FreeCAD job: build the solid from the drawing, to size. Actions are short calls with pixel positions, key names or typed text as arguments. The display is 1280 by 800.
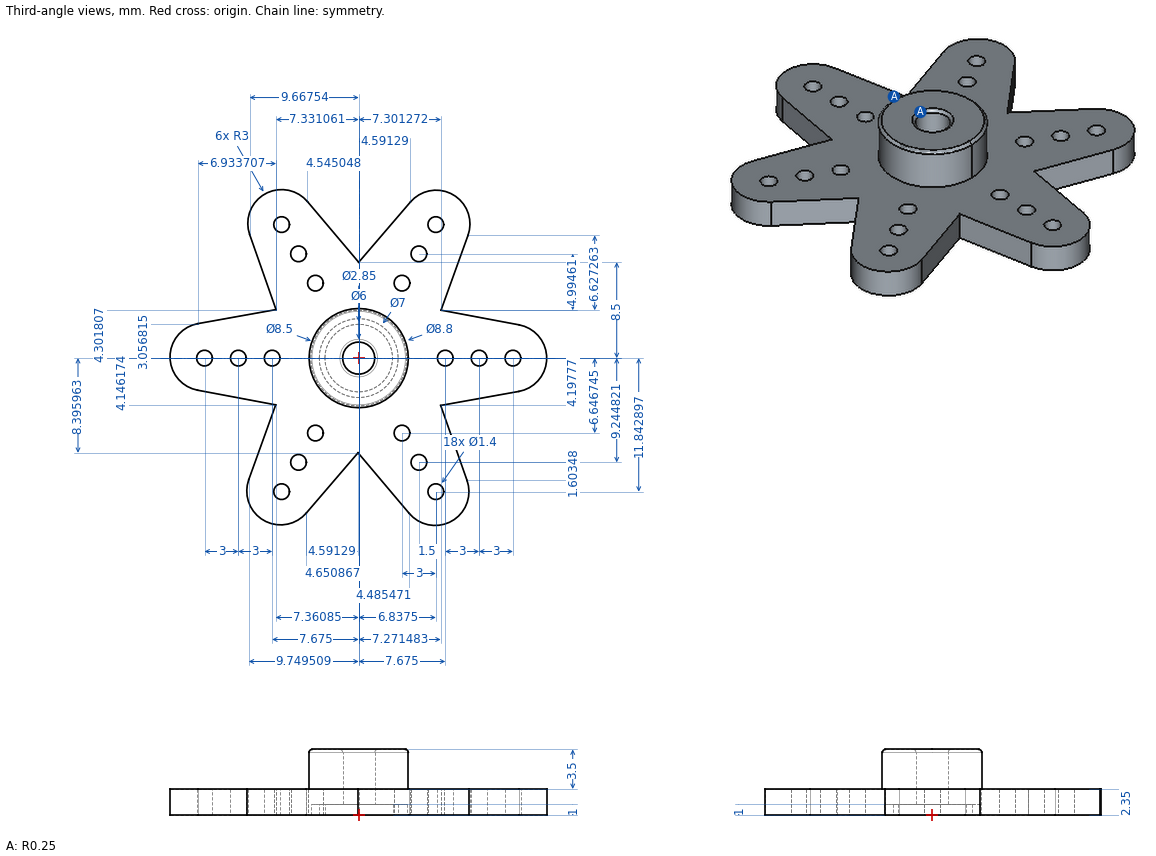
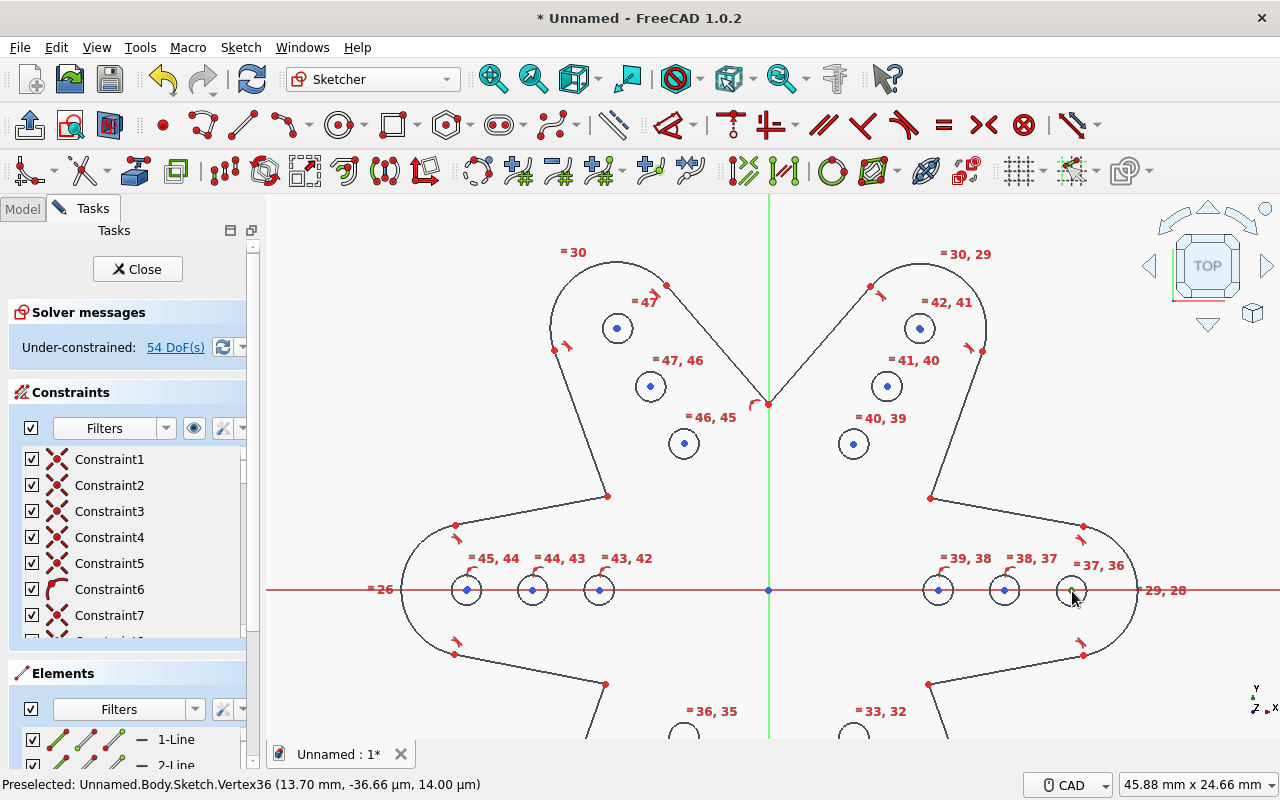
click(353, 590)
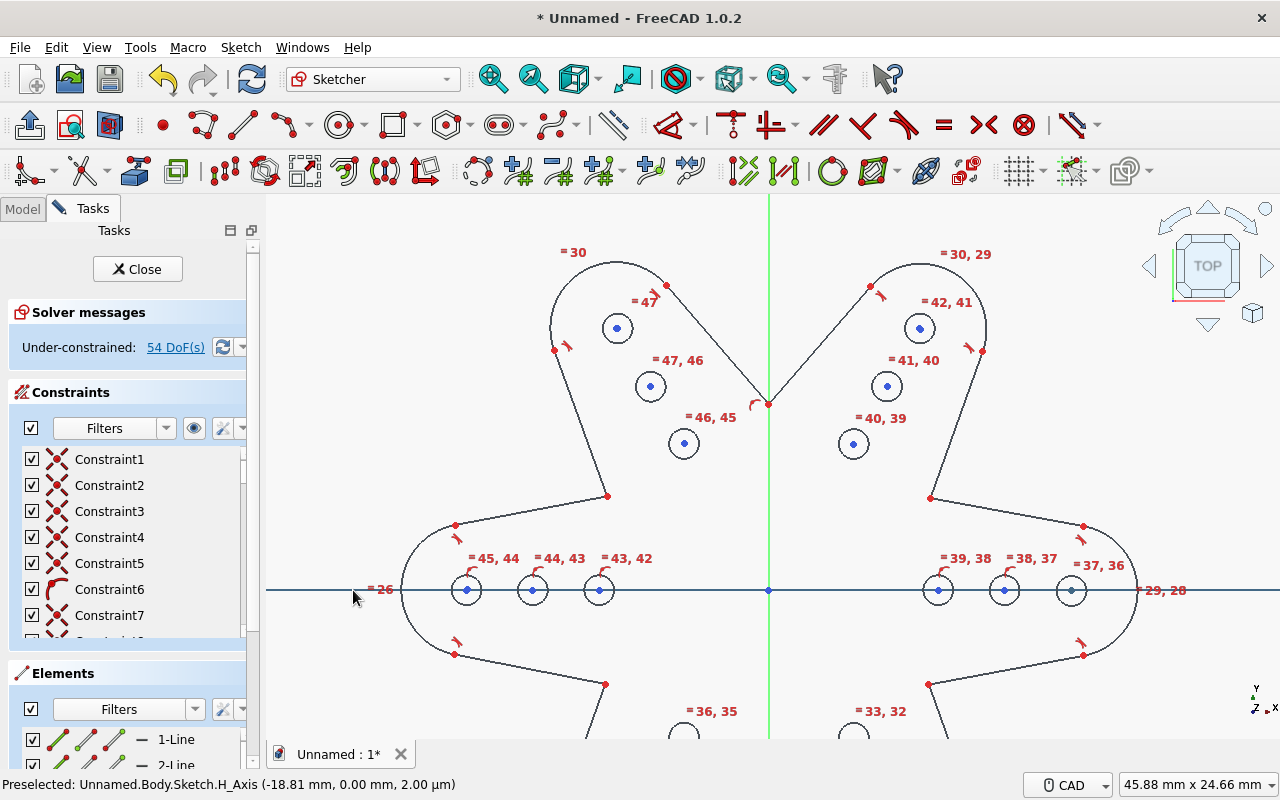
click(732, 126)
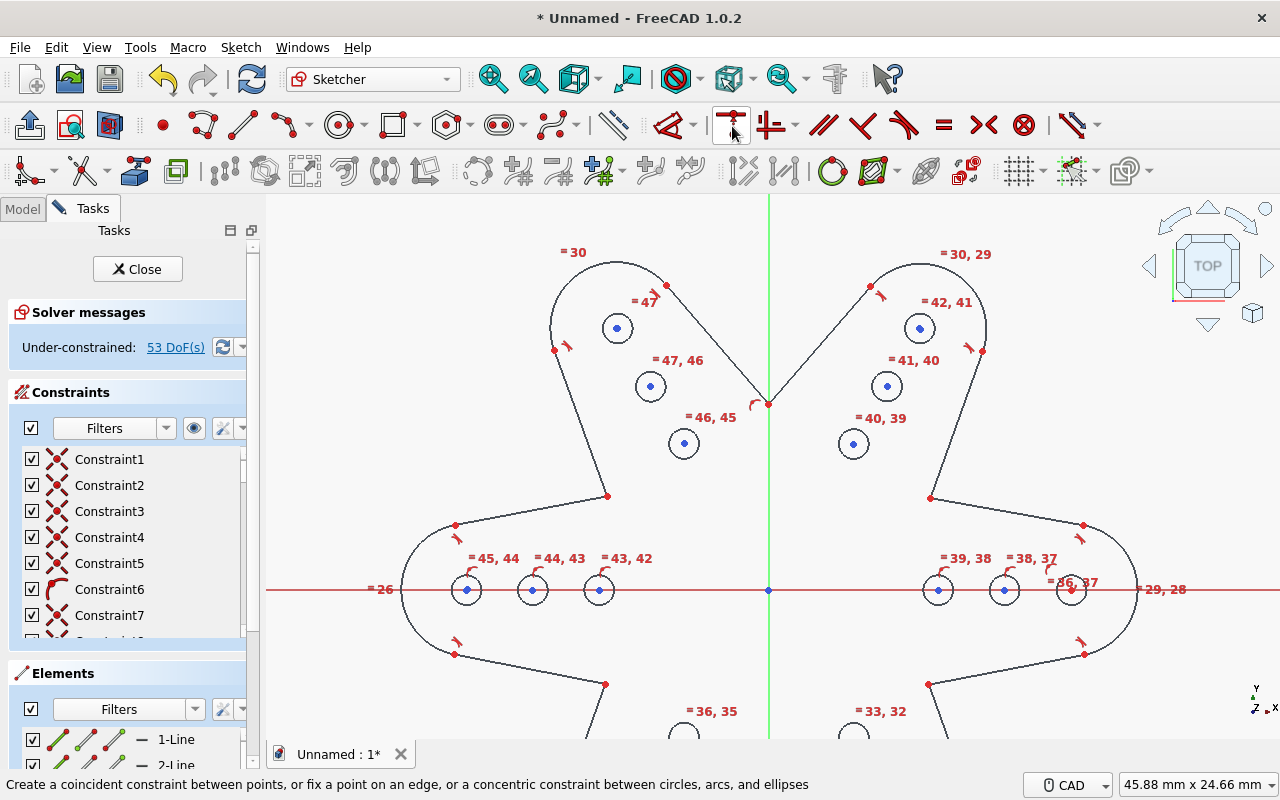
scroll(627, 317, down, 3)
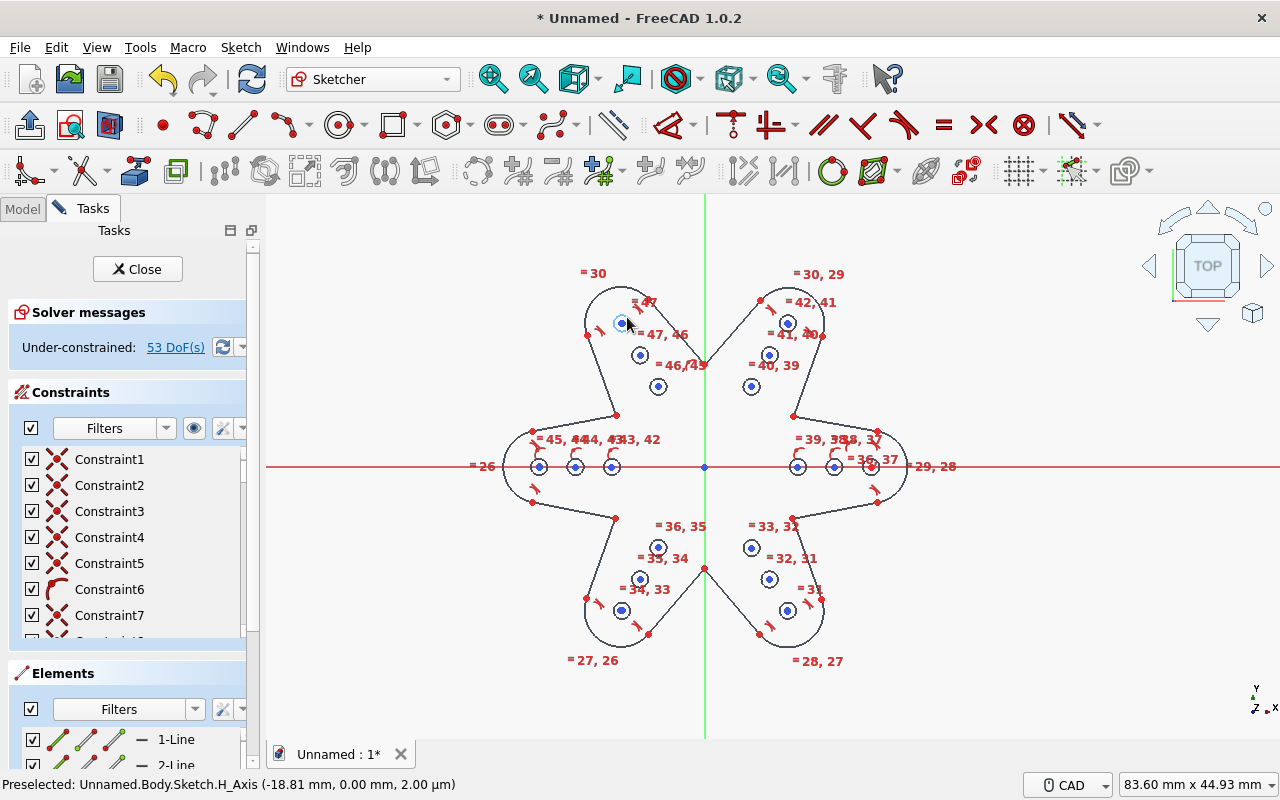
scroll(788, 611, up, 14)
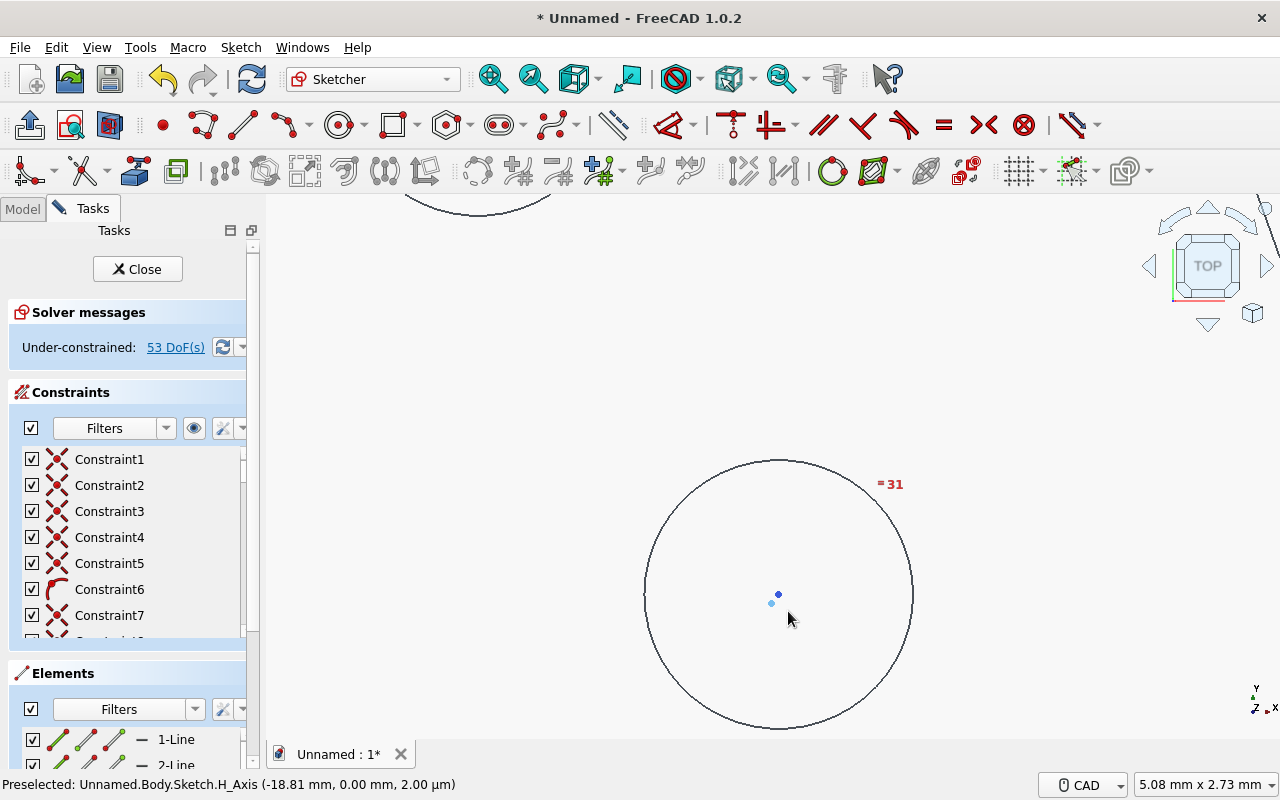
click(779, 594)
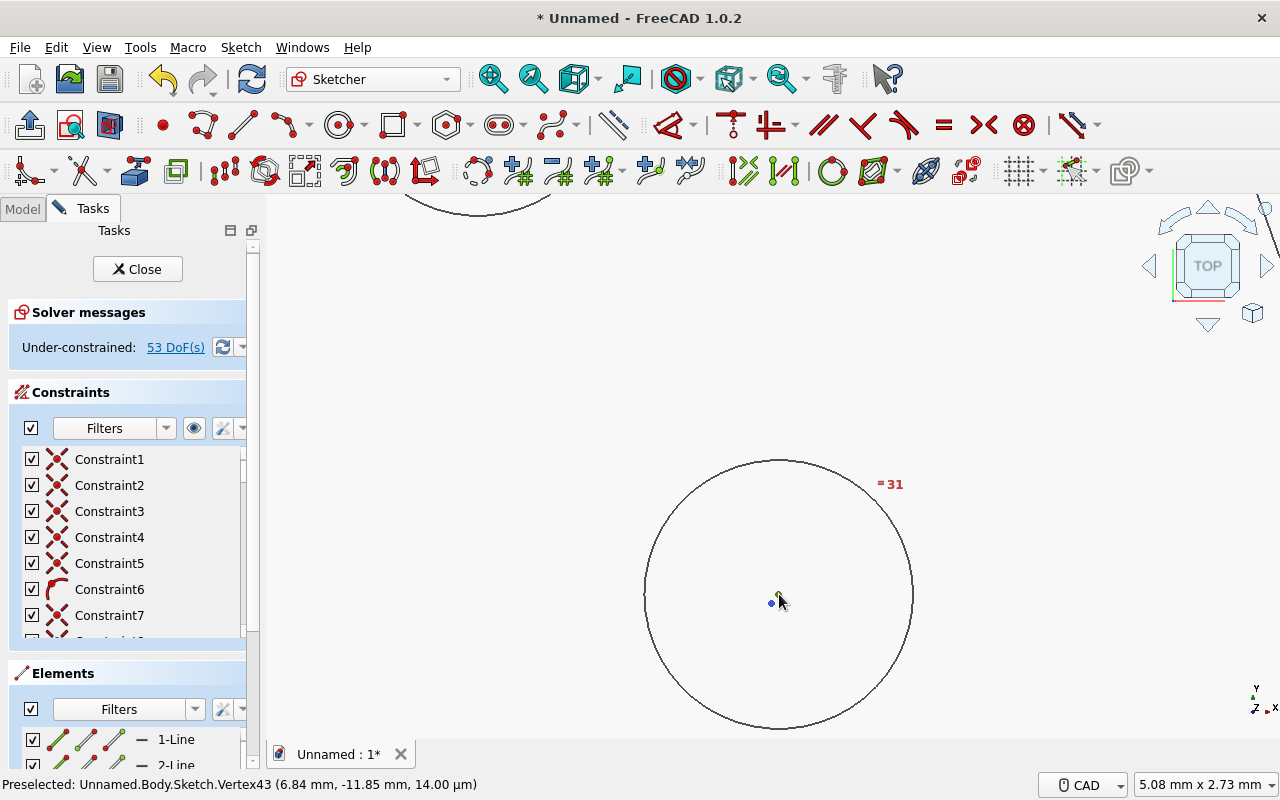
scroll(788, 612, down, 14)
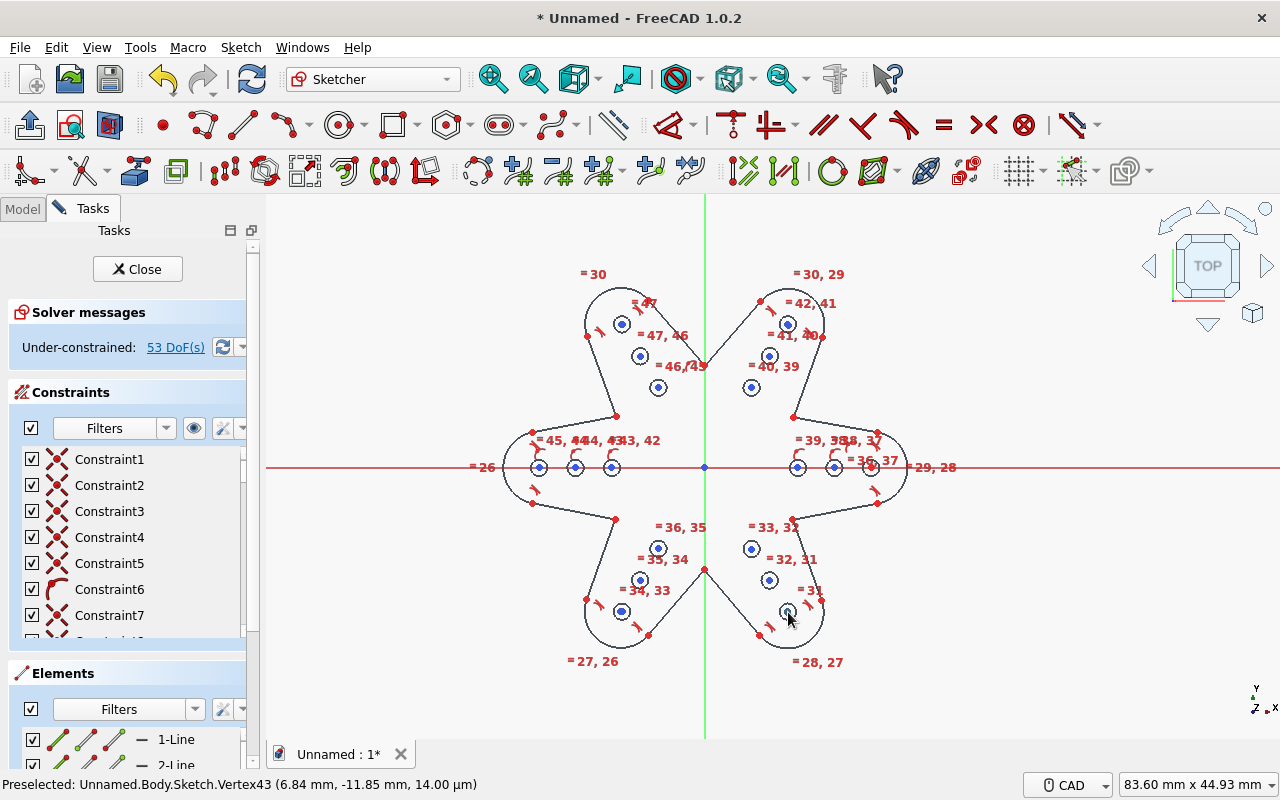
scroll(622, 612, up, 12)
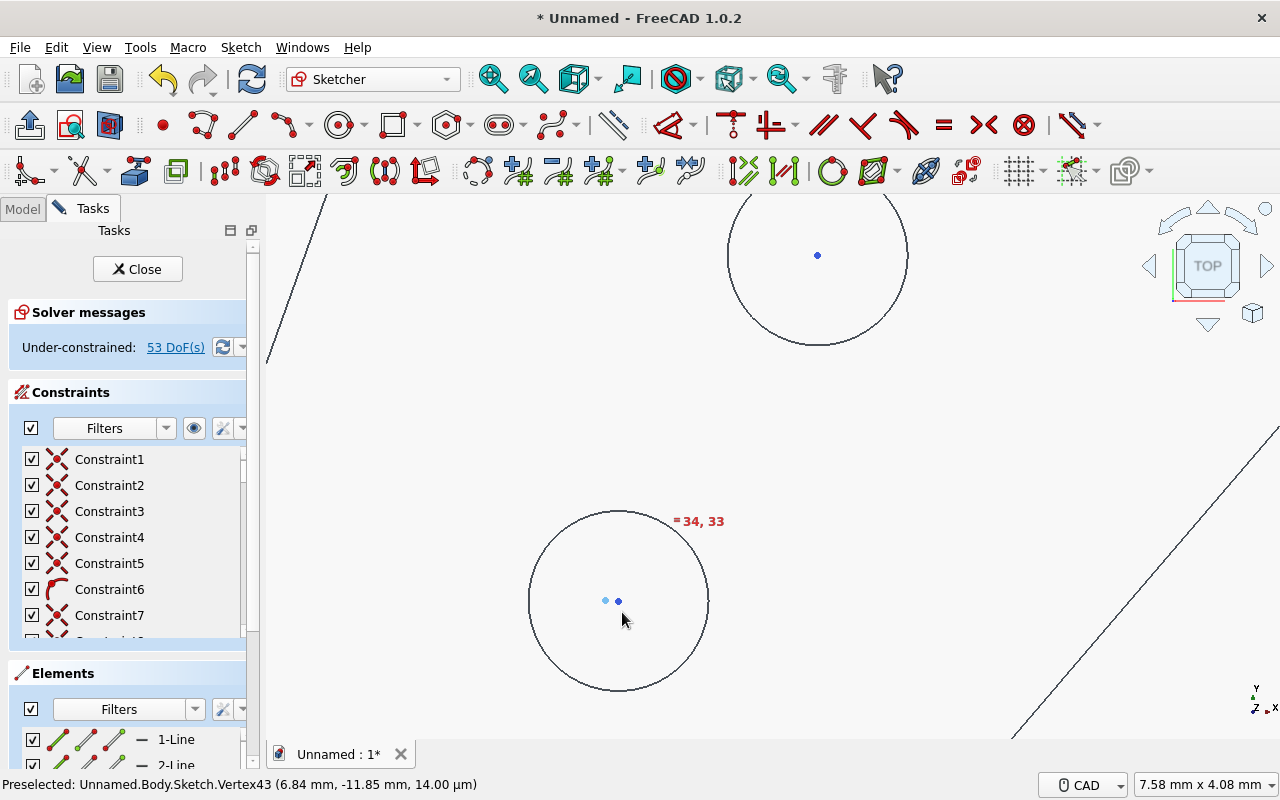
click(619, 601)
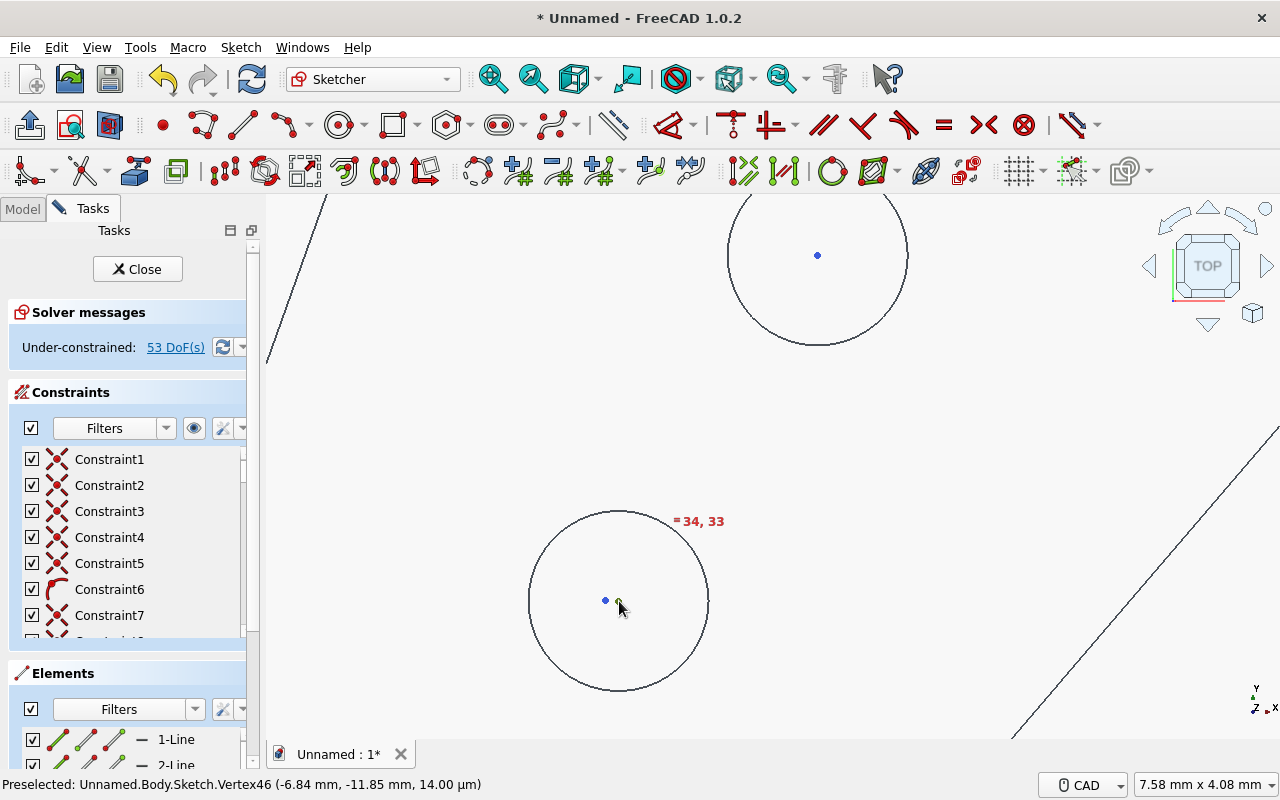
scroll(622, 612, down, 12)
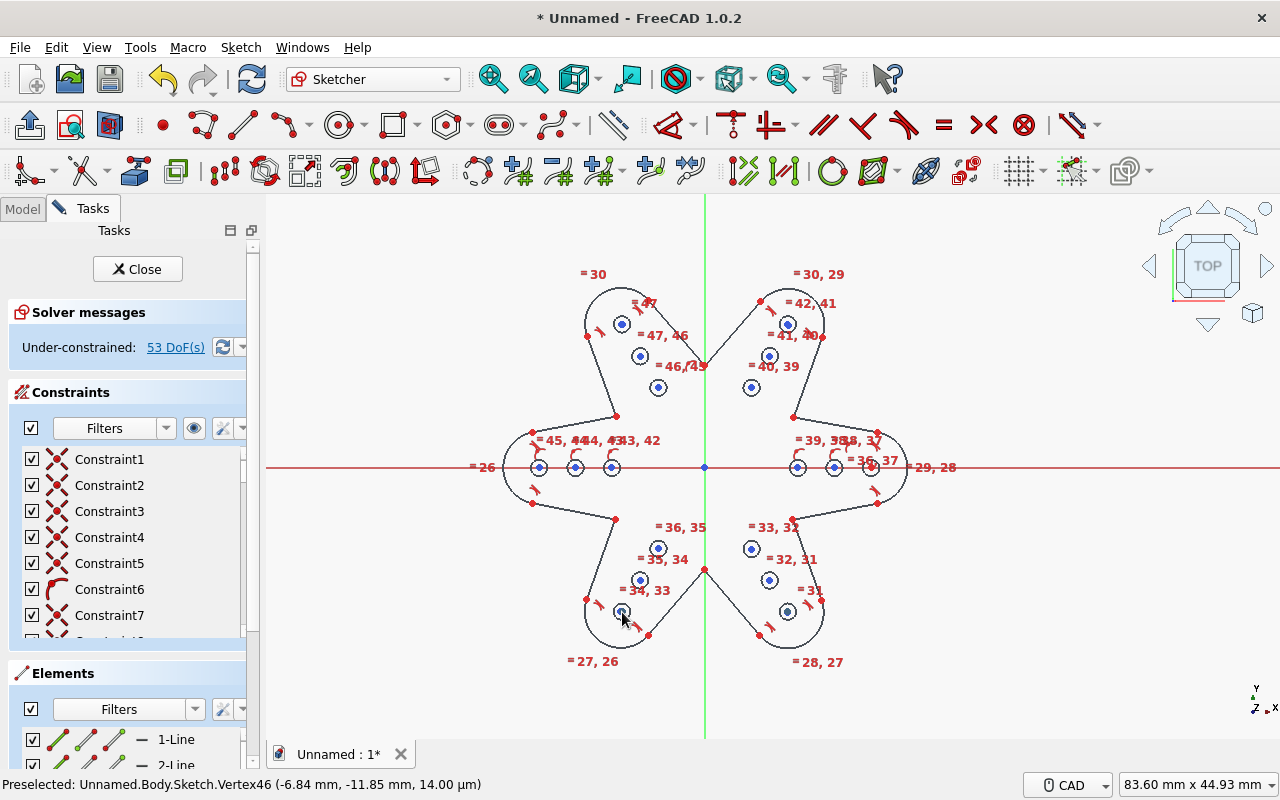
click(705, 676)